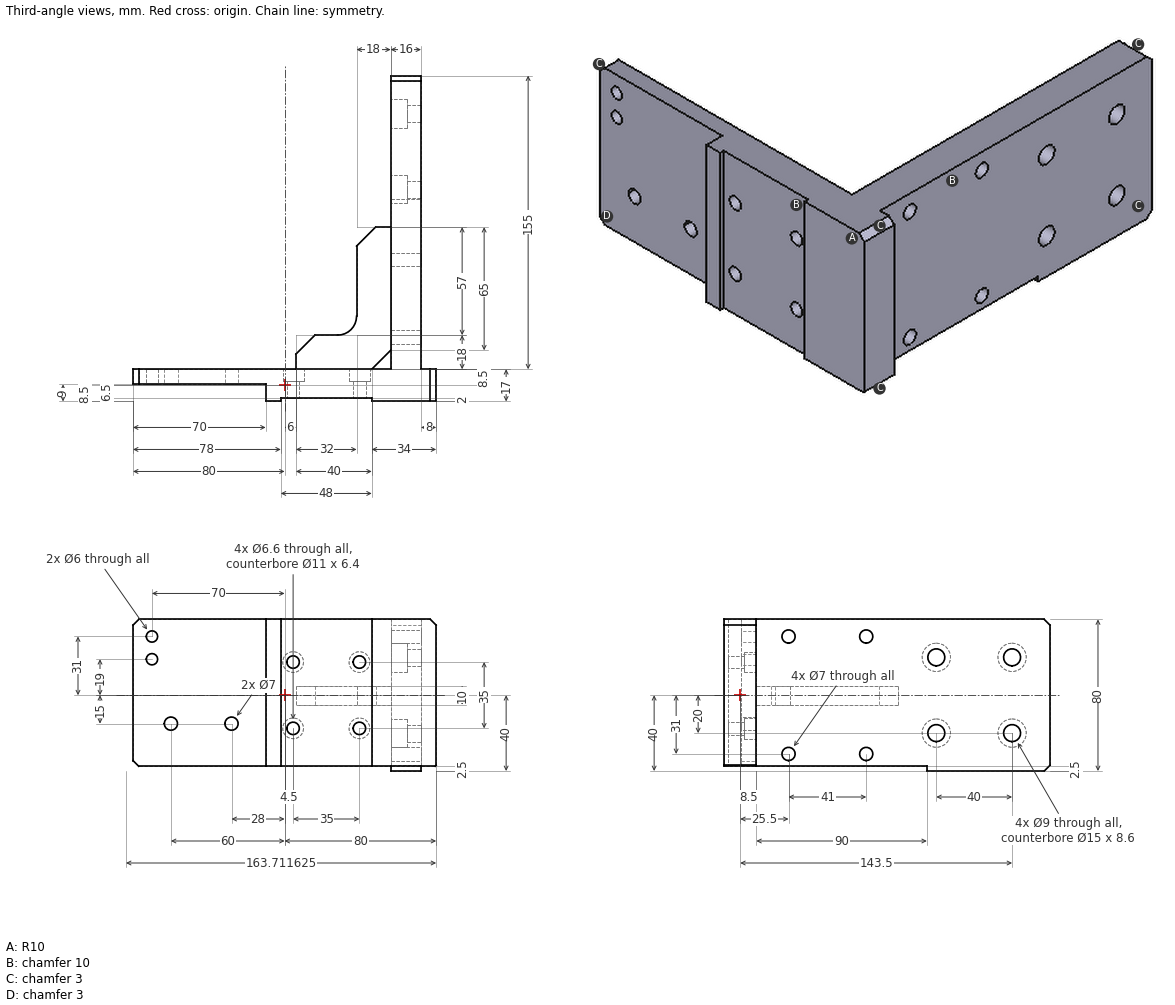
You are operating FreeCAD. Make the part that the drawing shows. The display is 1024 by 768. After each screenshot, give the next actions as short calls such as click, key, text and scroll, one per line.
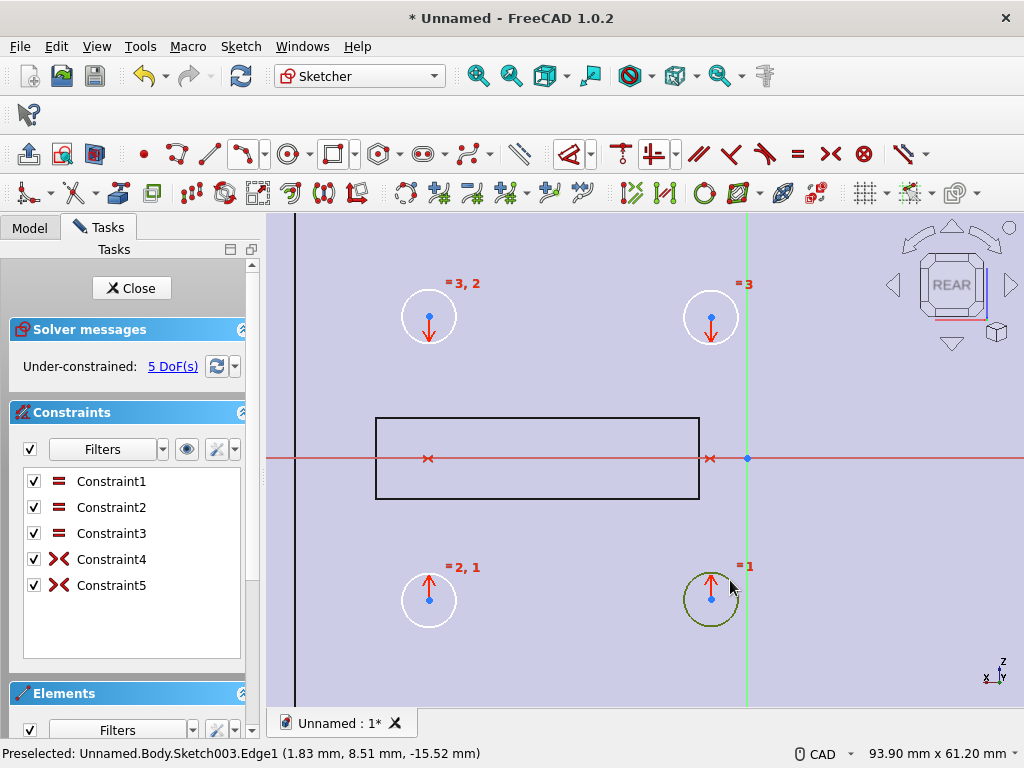
click(590, 154)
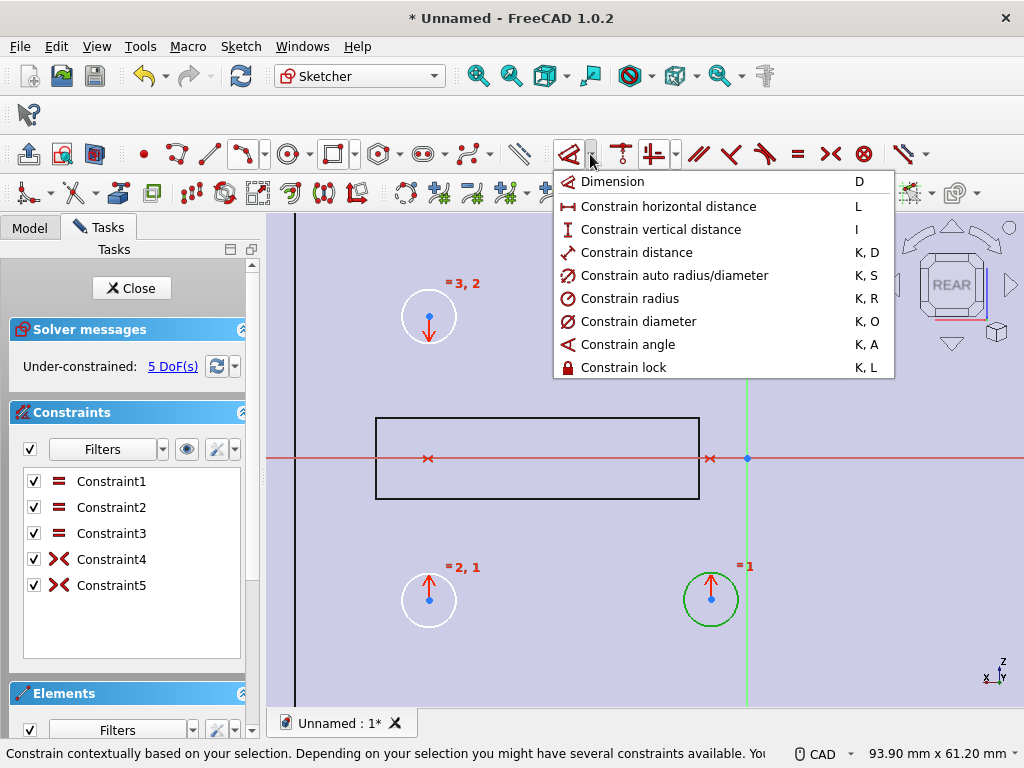
click(724, 322)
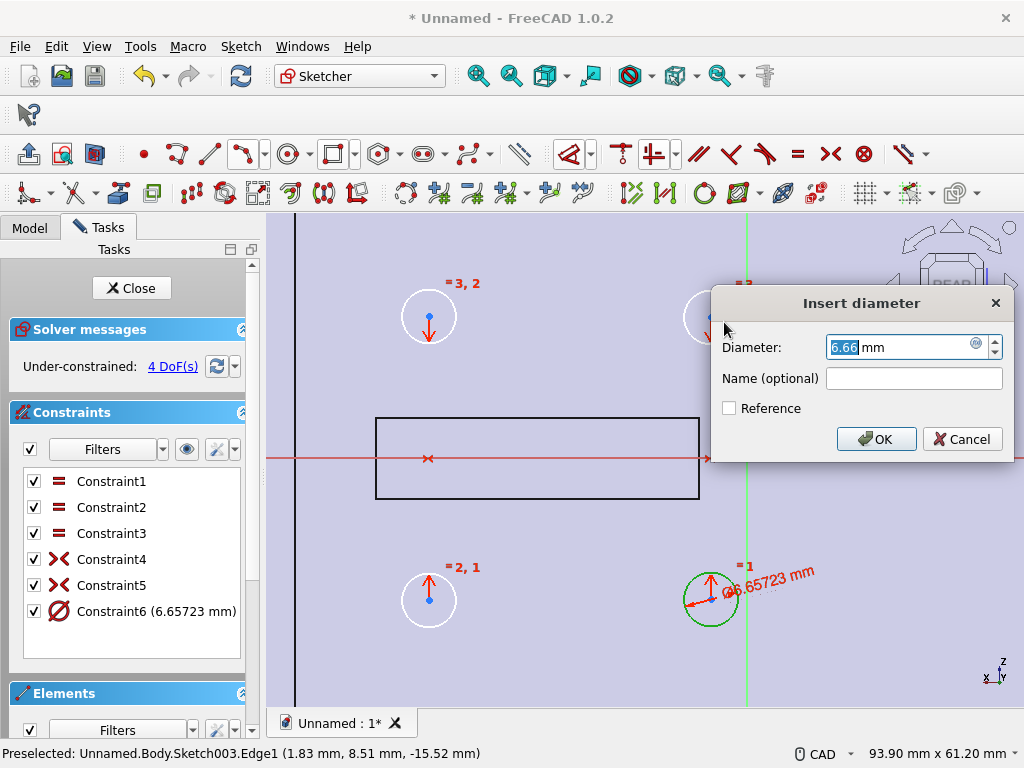
text(6.6)
key(Return)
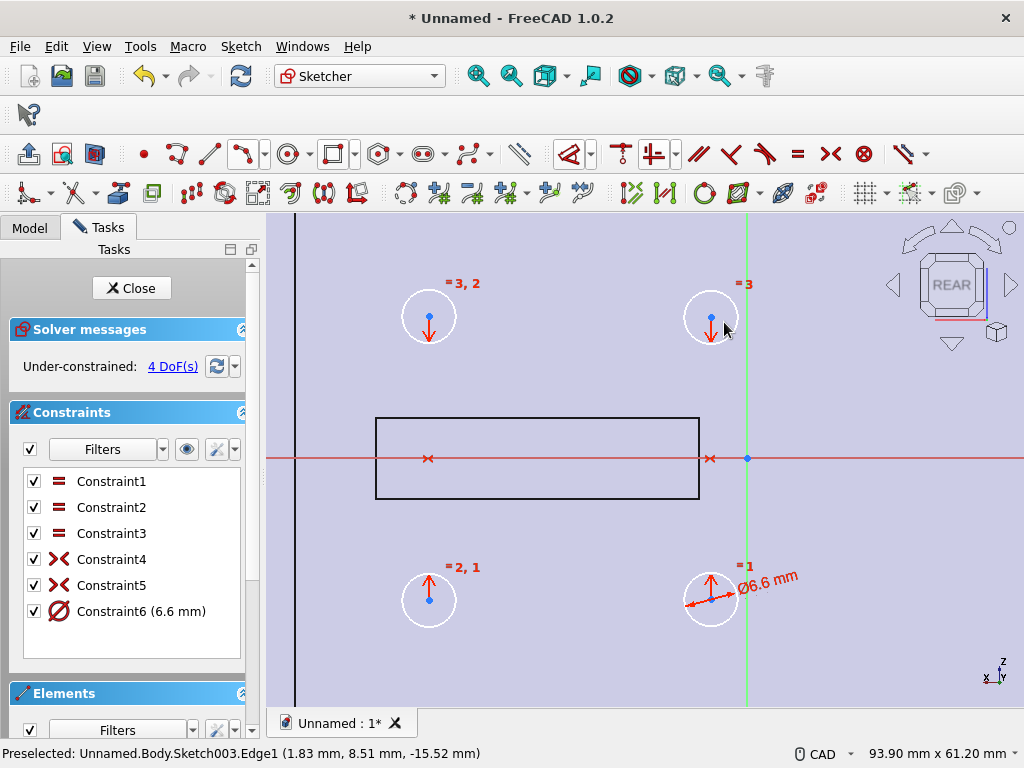
click(711, 600)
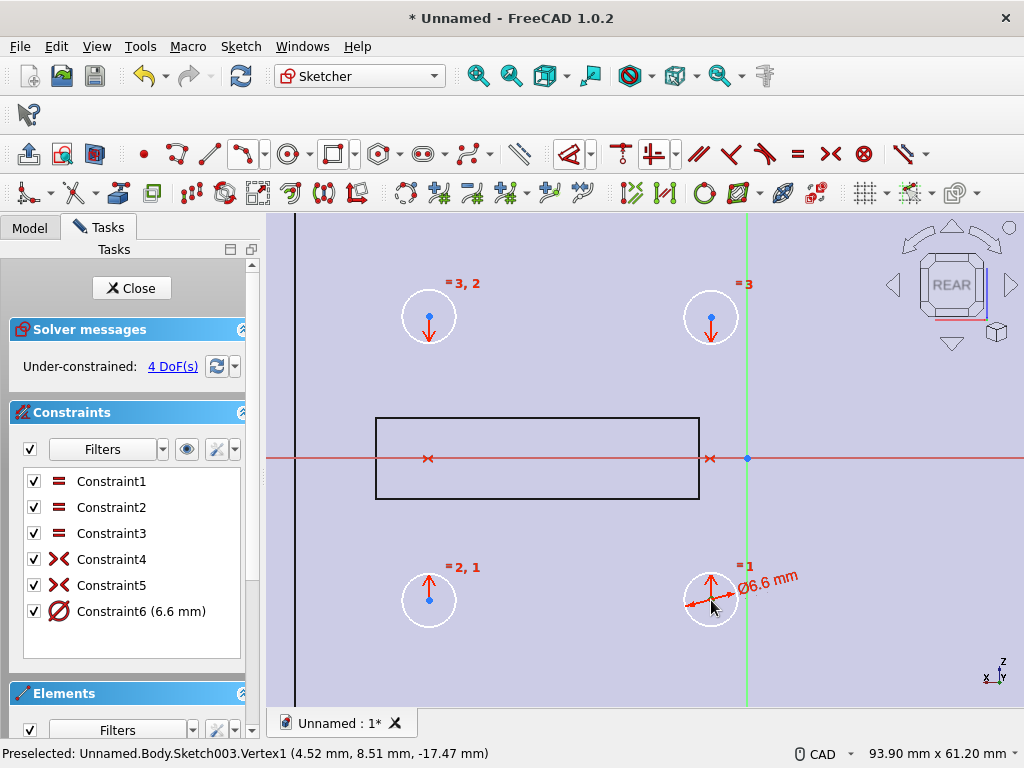
key(l)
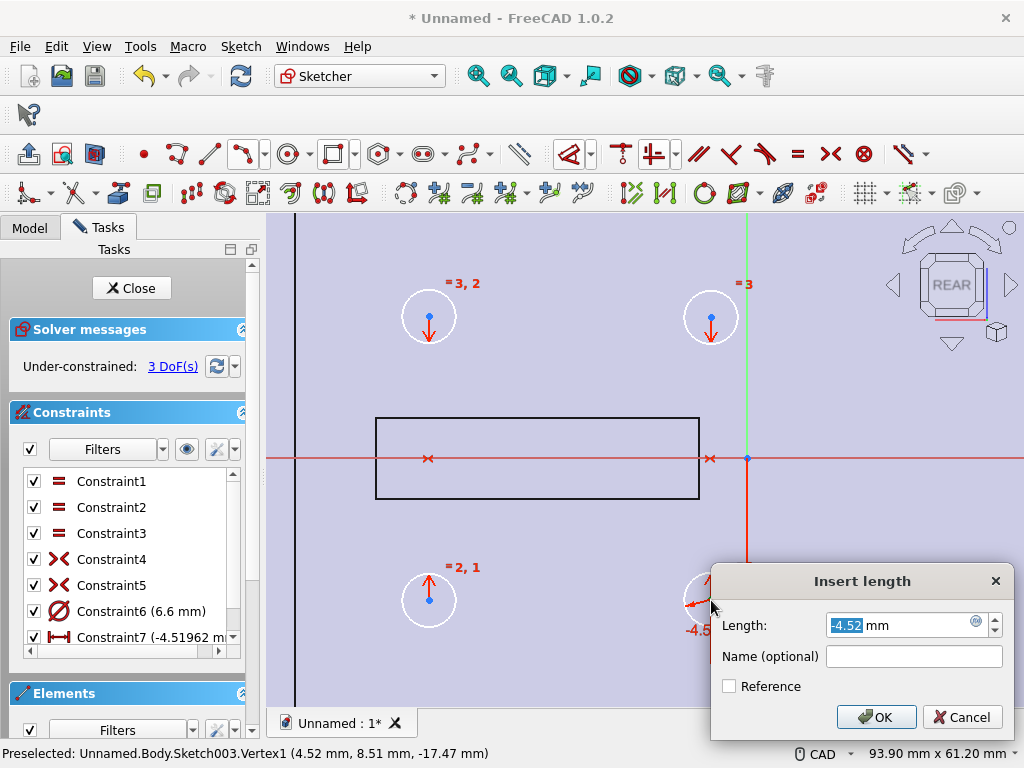
text(-4.5)
key(Return)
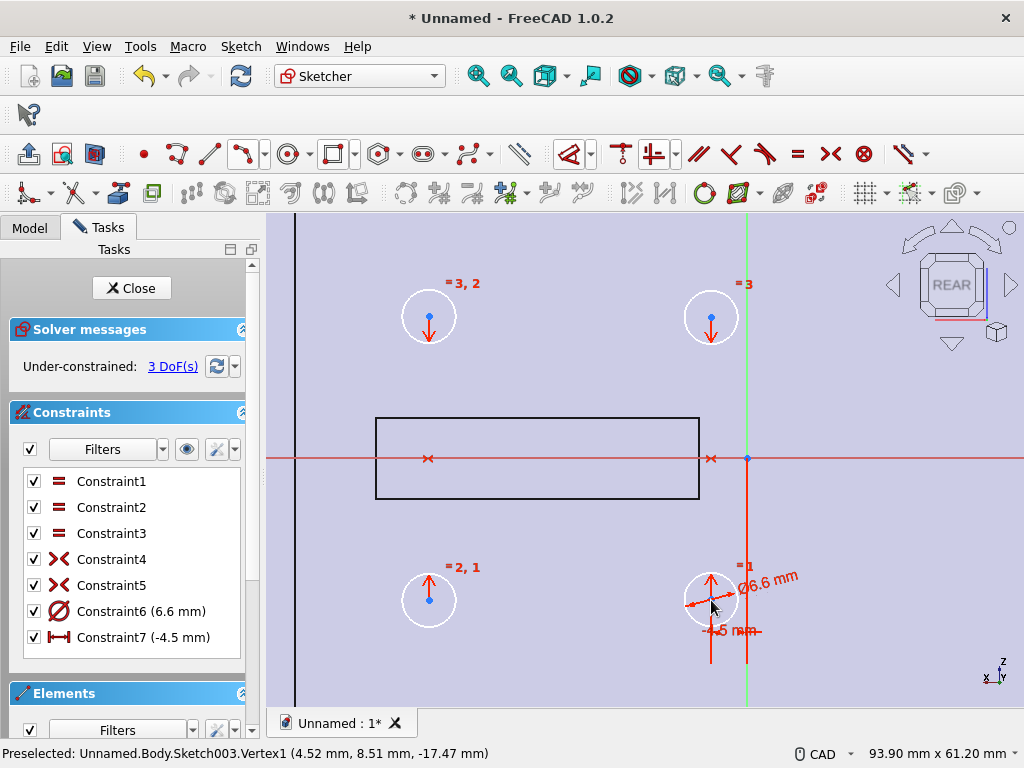
click(711, 600)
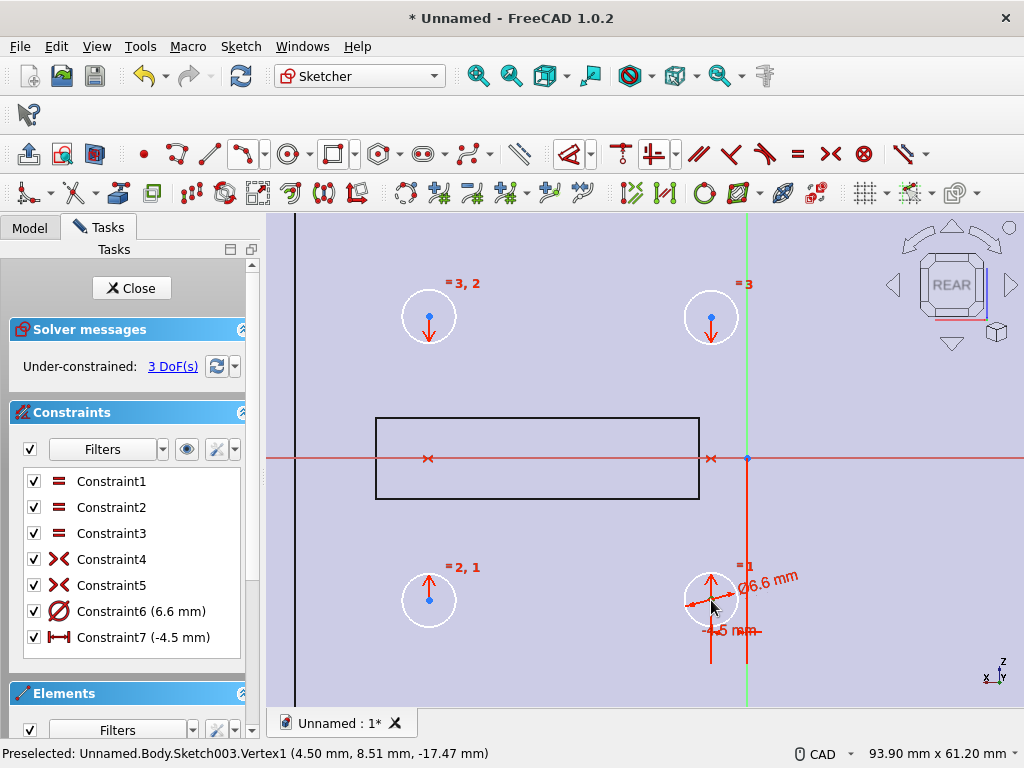
click(429, 600)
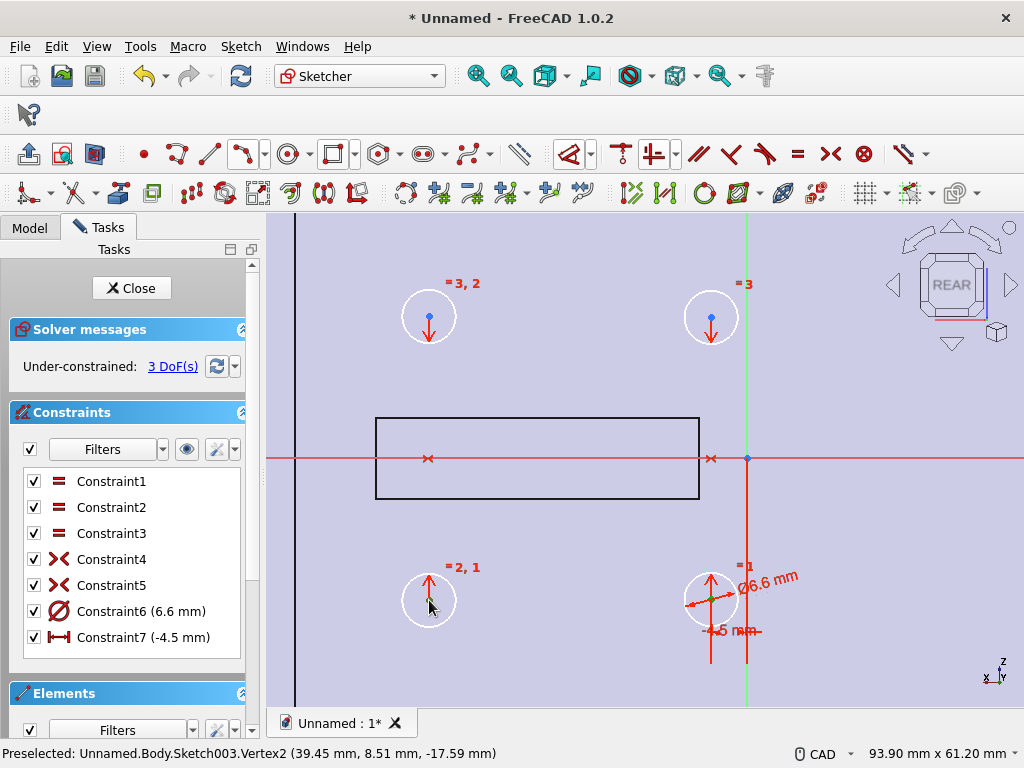
click(590, 154)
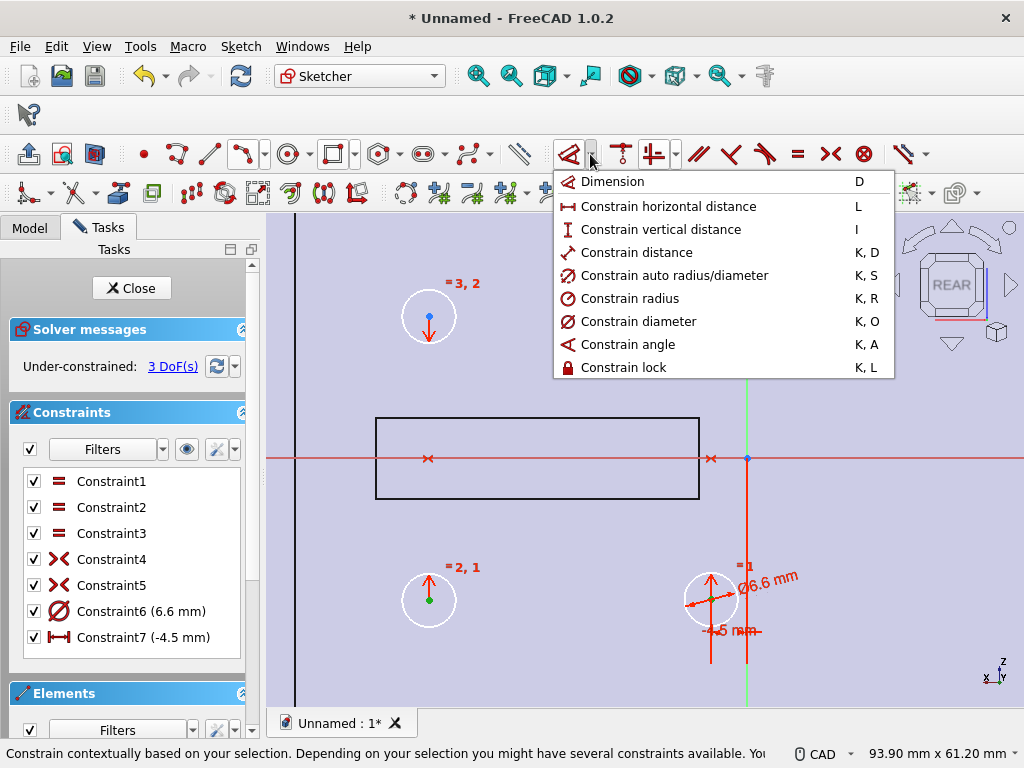
click(724, 206)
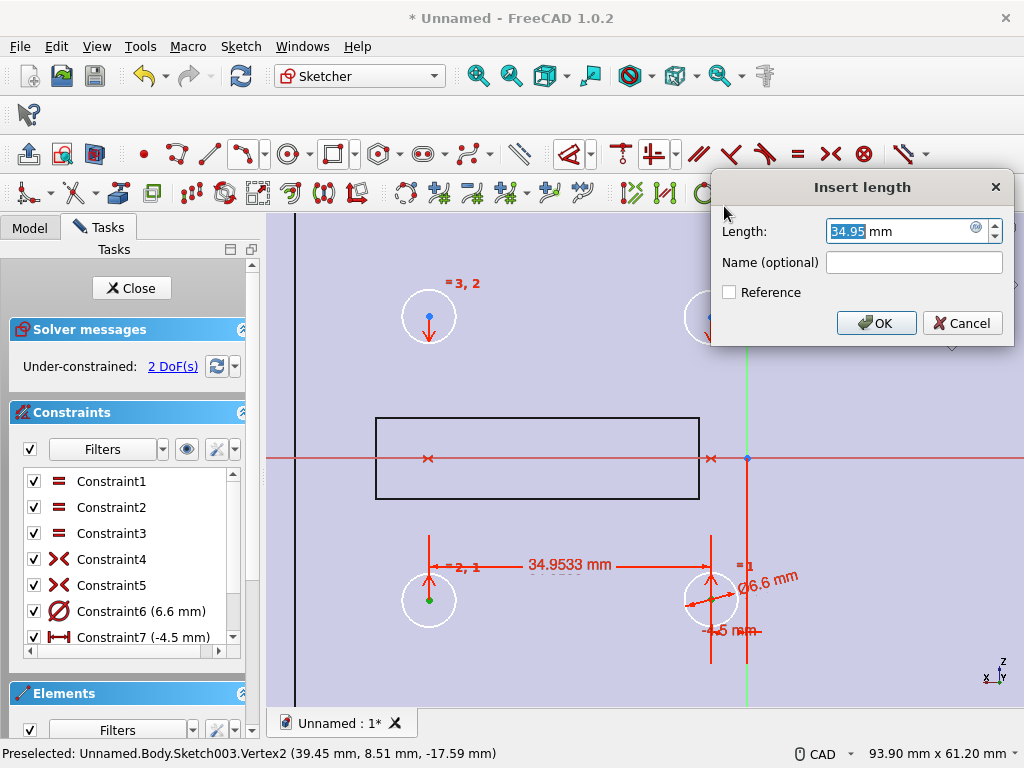
text(35)
key(Return)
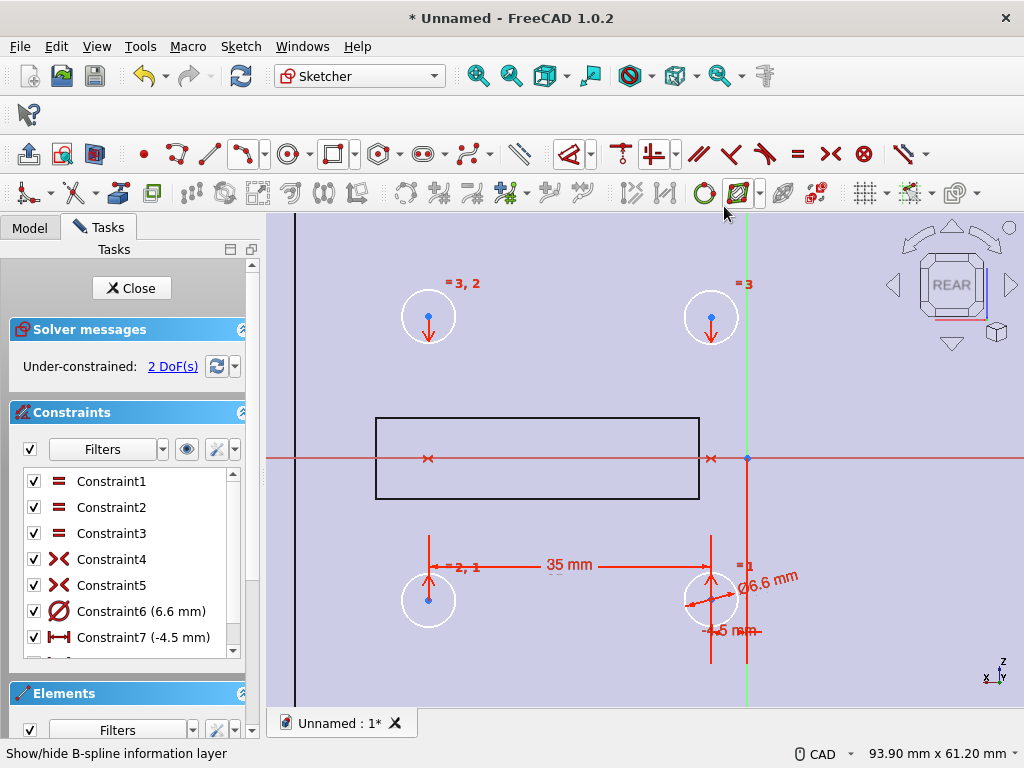
click(429, 600)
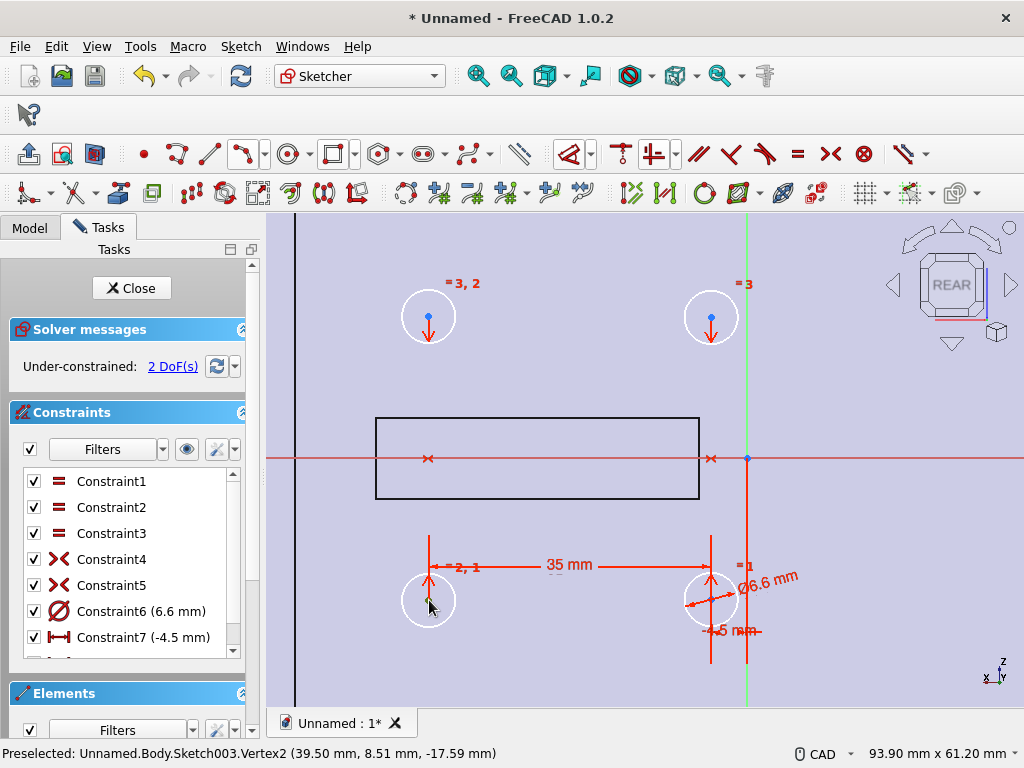
click(429, 317)